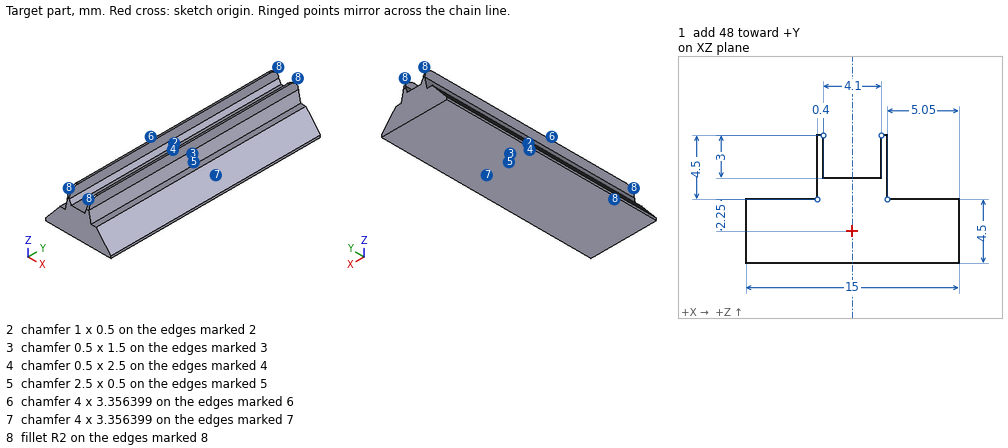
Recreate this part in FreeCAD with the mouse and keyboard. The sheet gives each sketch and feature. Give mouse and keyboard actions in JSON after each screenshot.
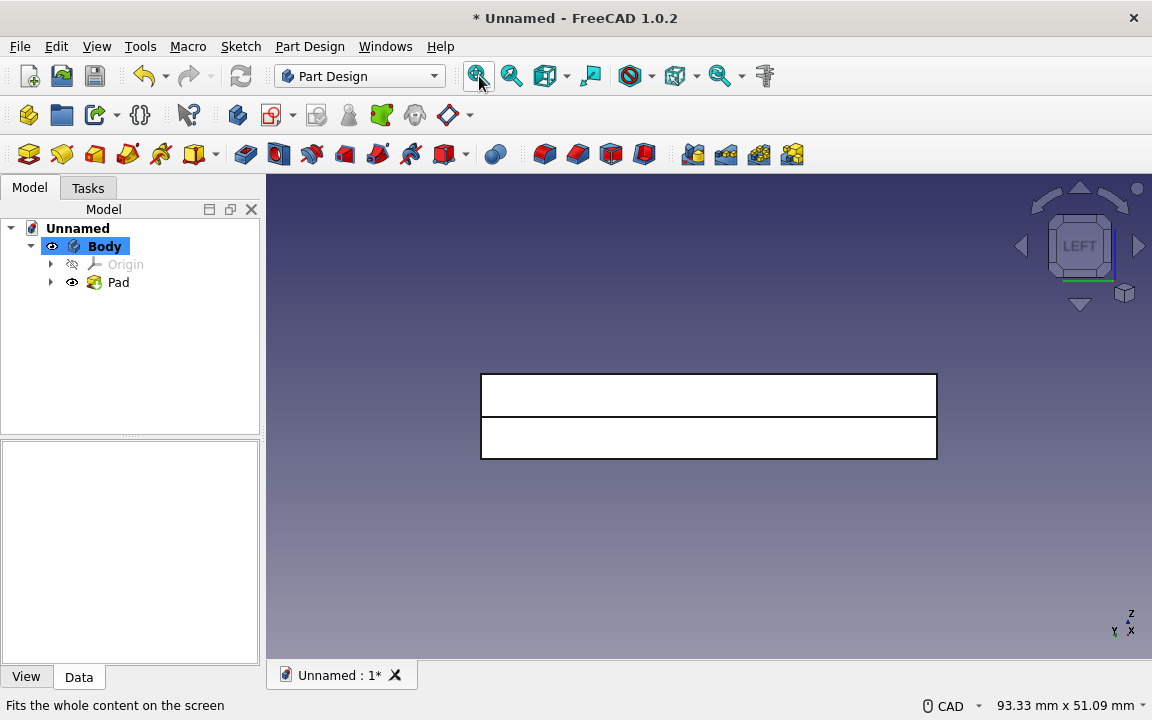
{"action": "key", "text": "v 3"}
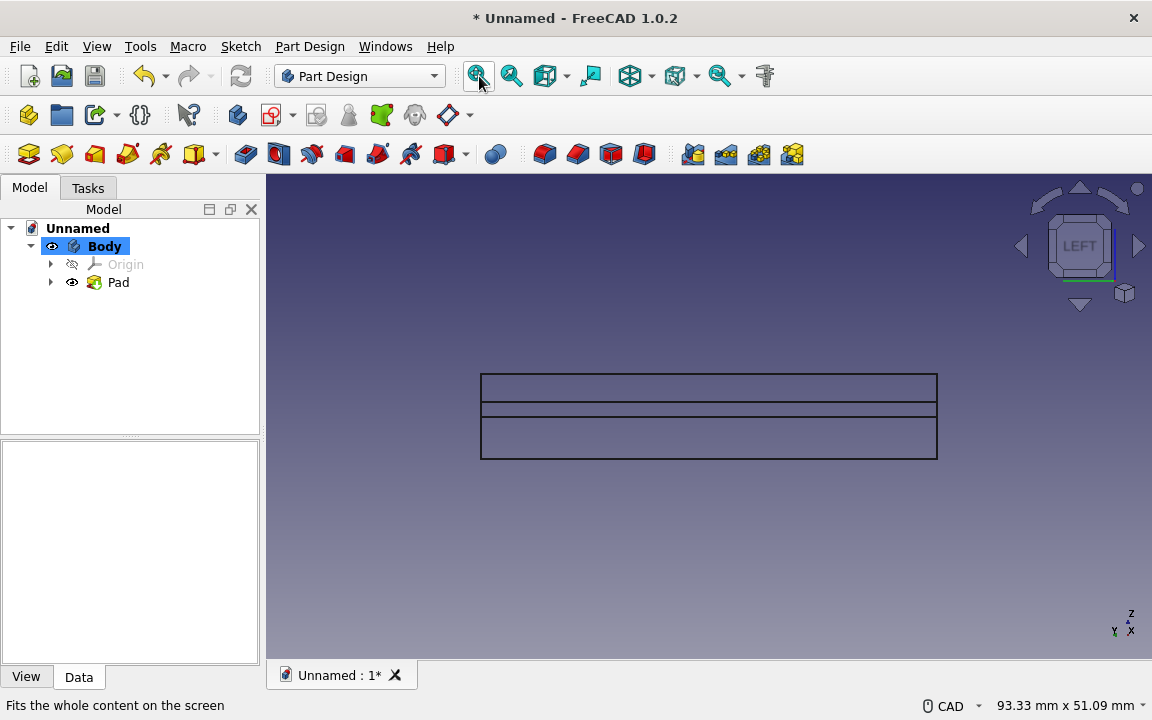
{"action": "key", "text": "0"}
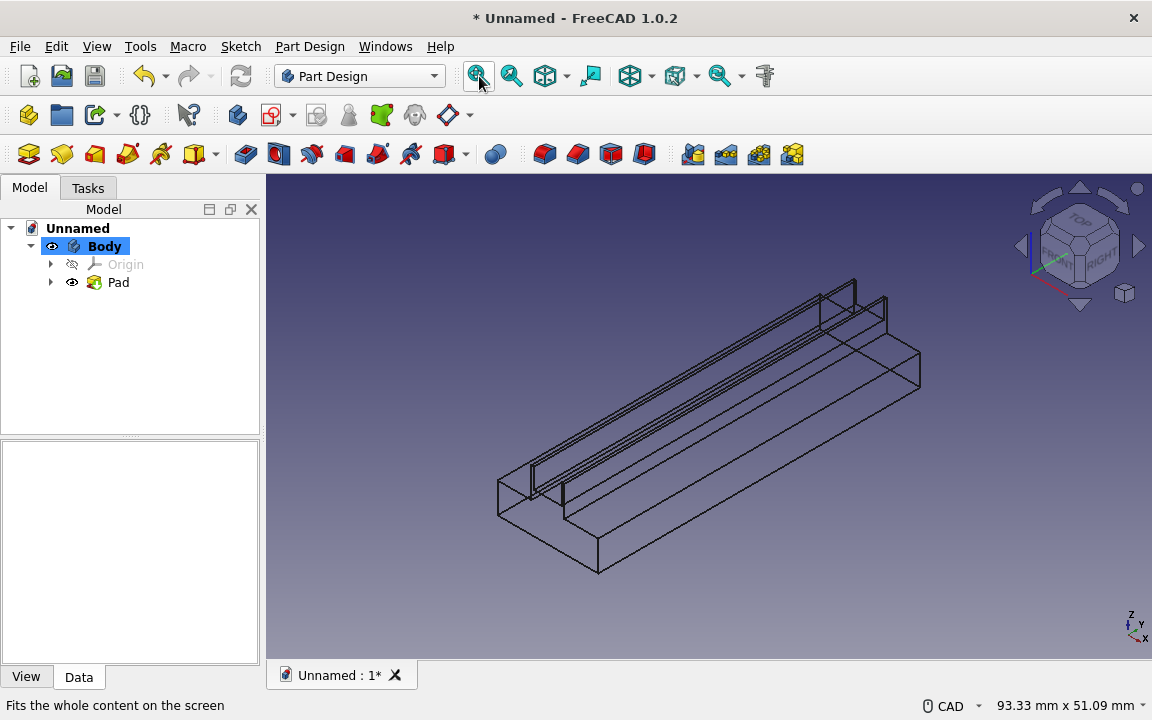
{"action": "left_click", "coordinate": [695, 396]}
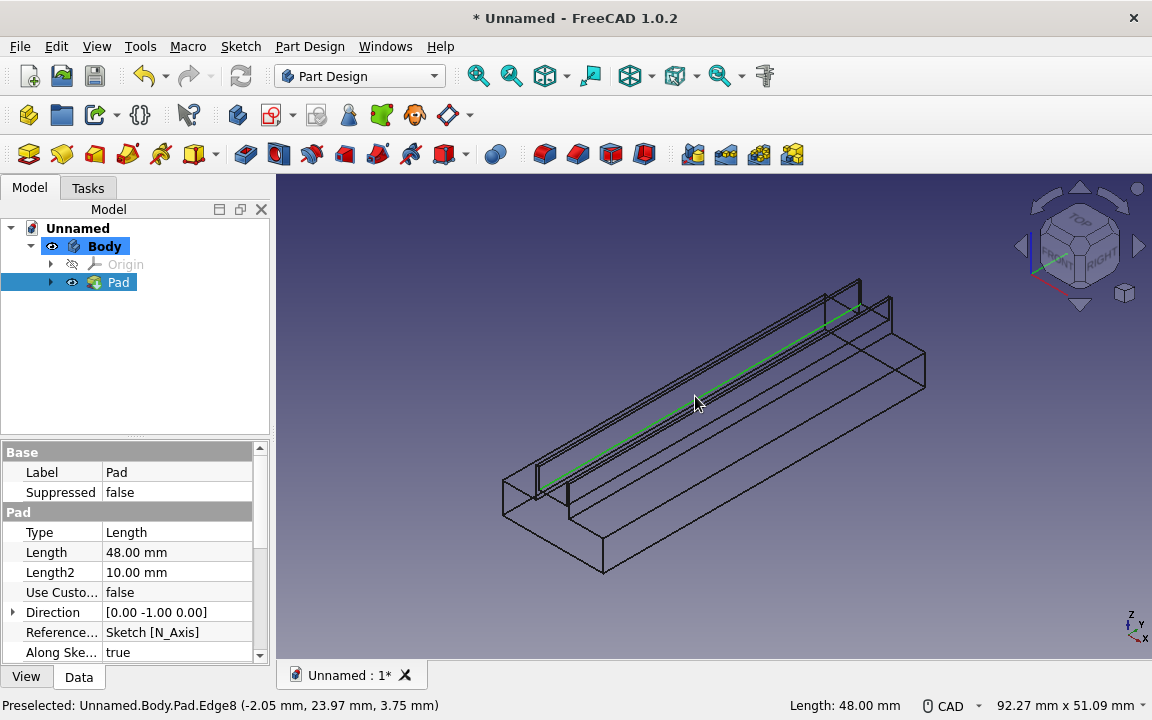
{"action": "key", "text": "v 1"}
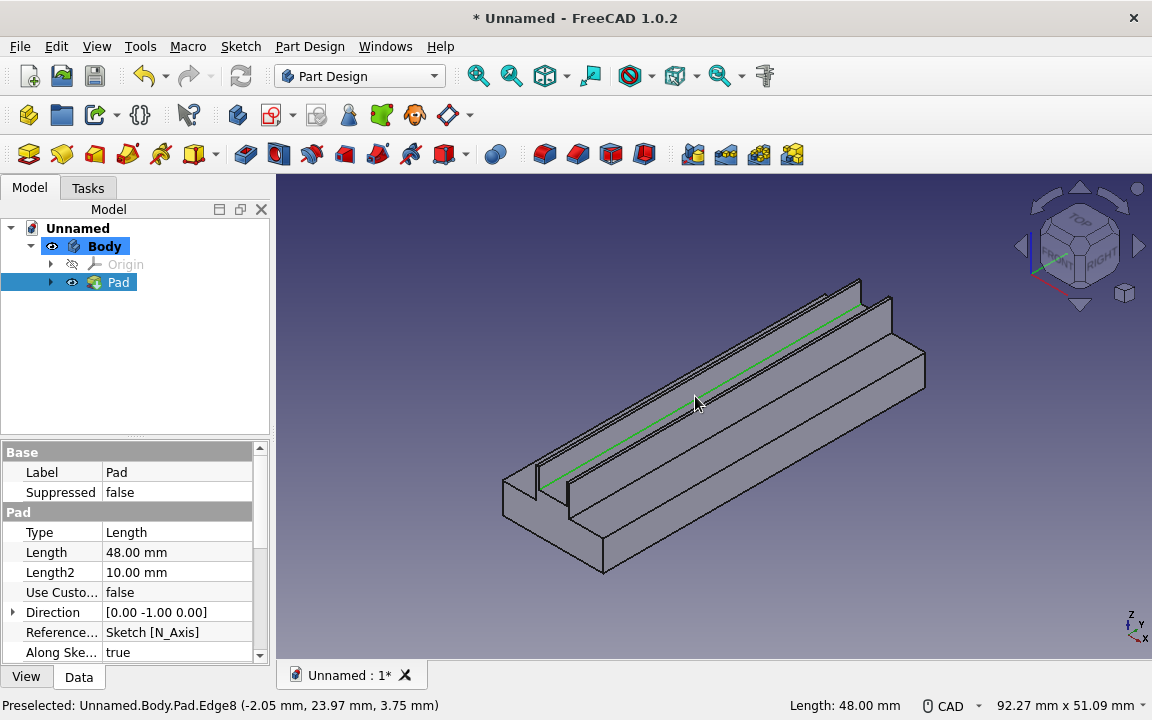
{"action": "left_click", "coordinate": [578, 154]}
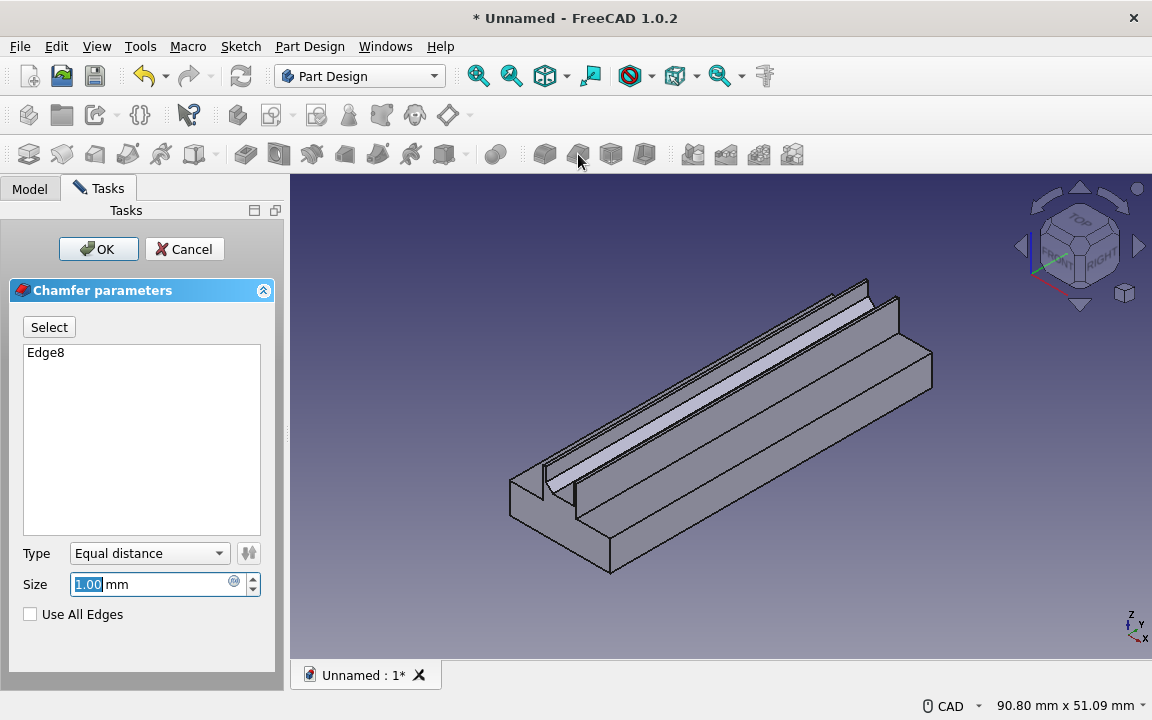
{"action": "type", "text": "1"}
{"action": "key", "text": "Tab"}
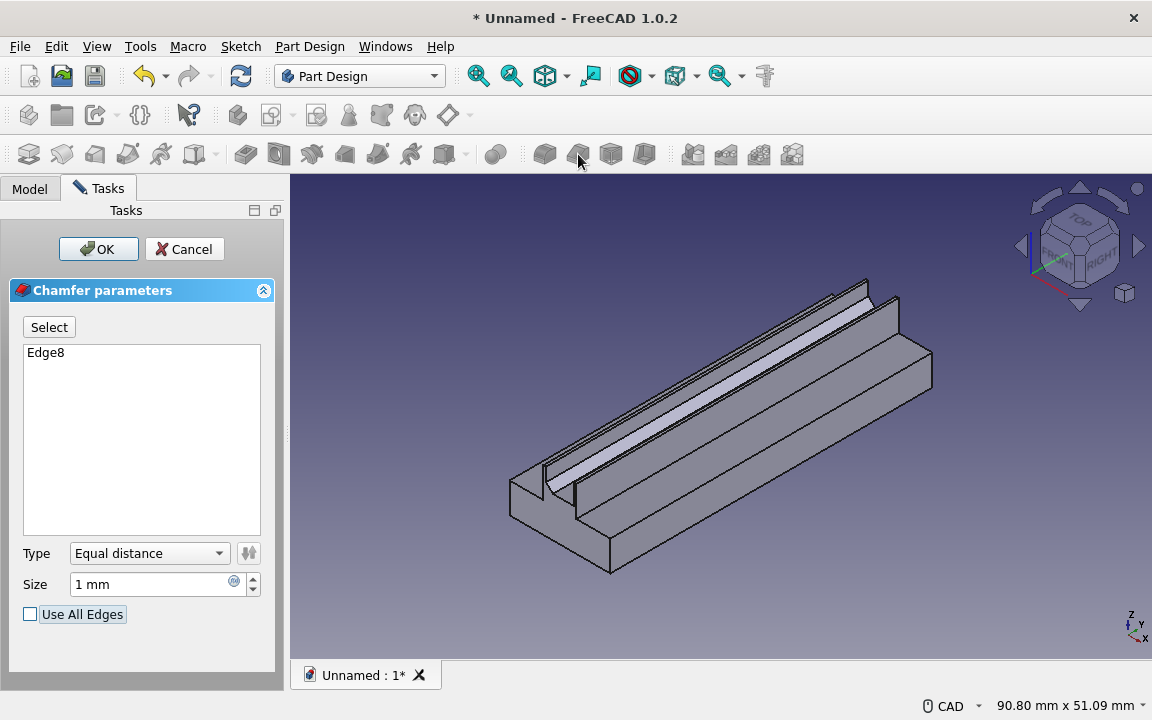
{"action": "left_click", "coordinate": [150, 554]}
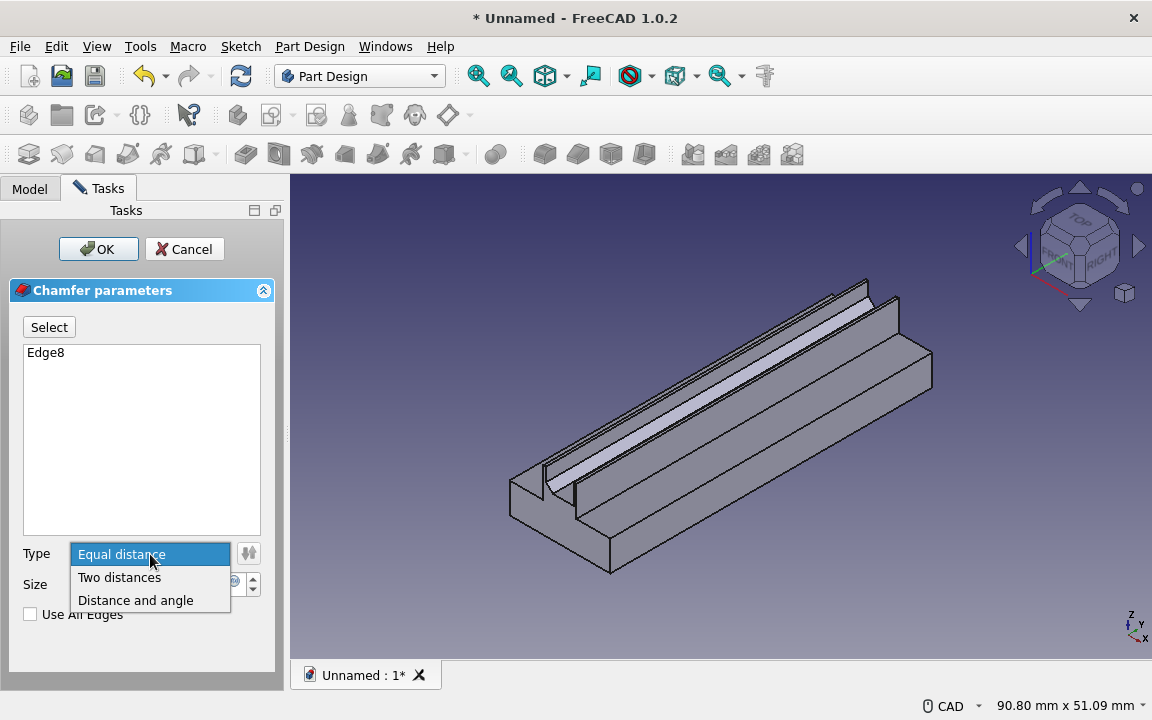
{"action": "left_click", "coordinate": [148, 578]}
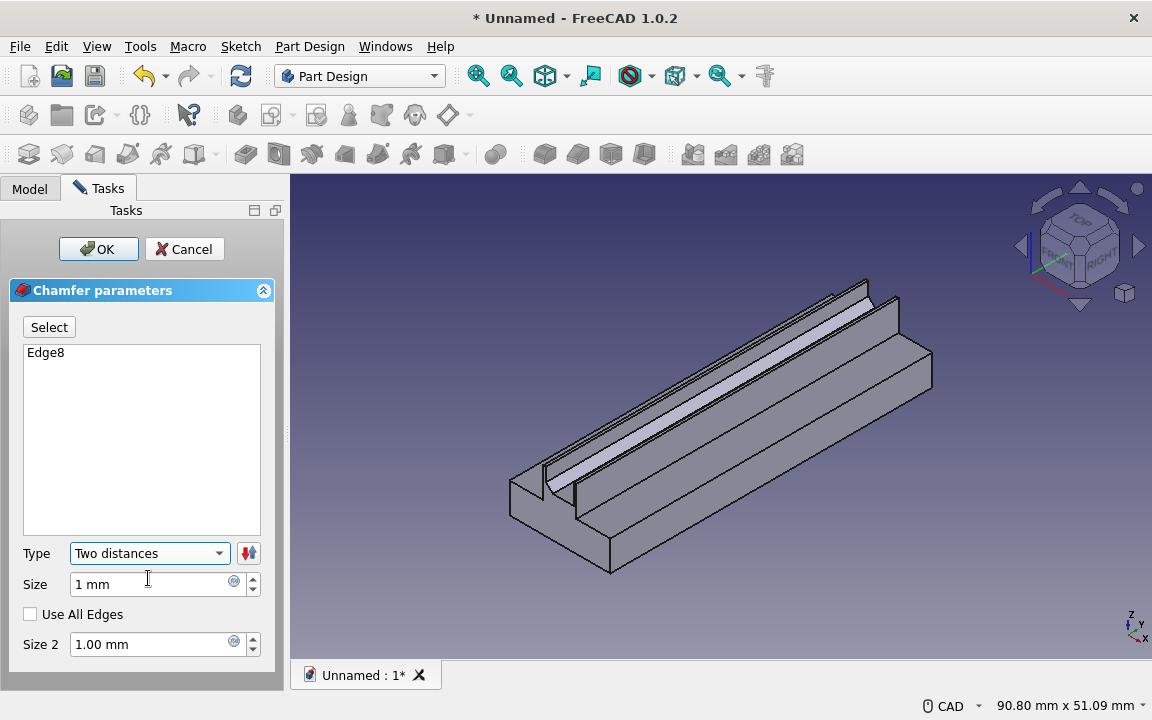
{"action": "triple_click", "coordinate": [158, 644]}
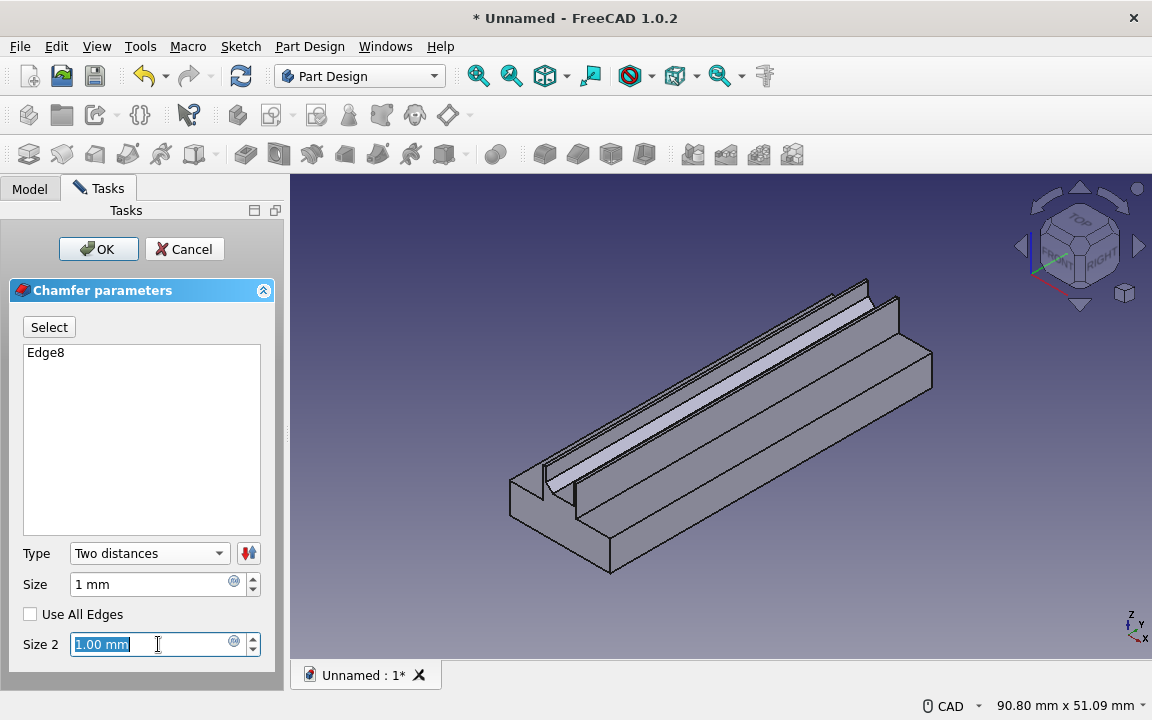
{"action": "type", "text": "0.5"}
{"action": "key", "text": "Tab"}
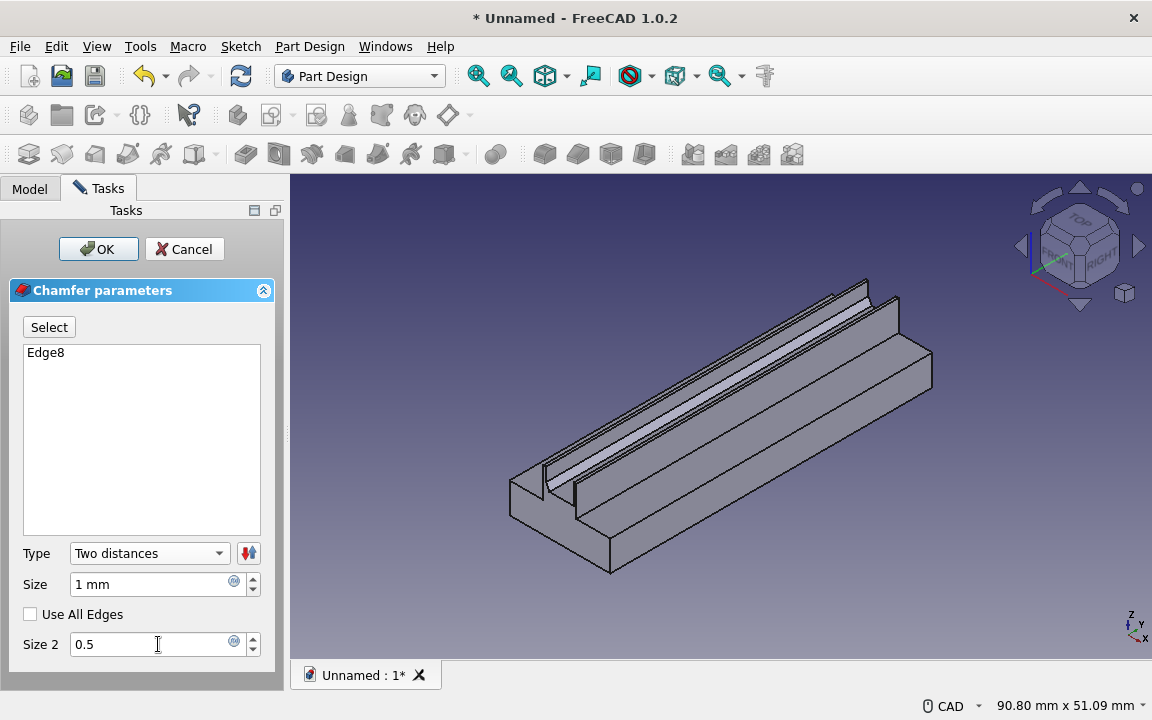
{"action": "left_click", "coordinate": [99, 249]}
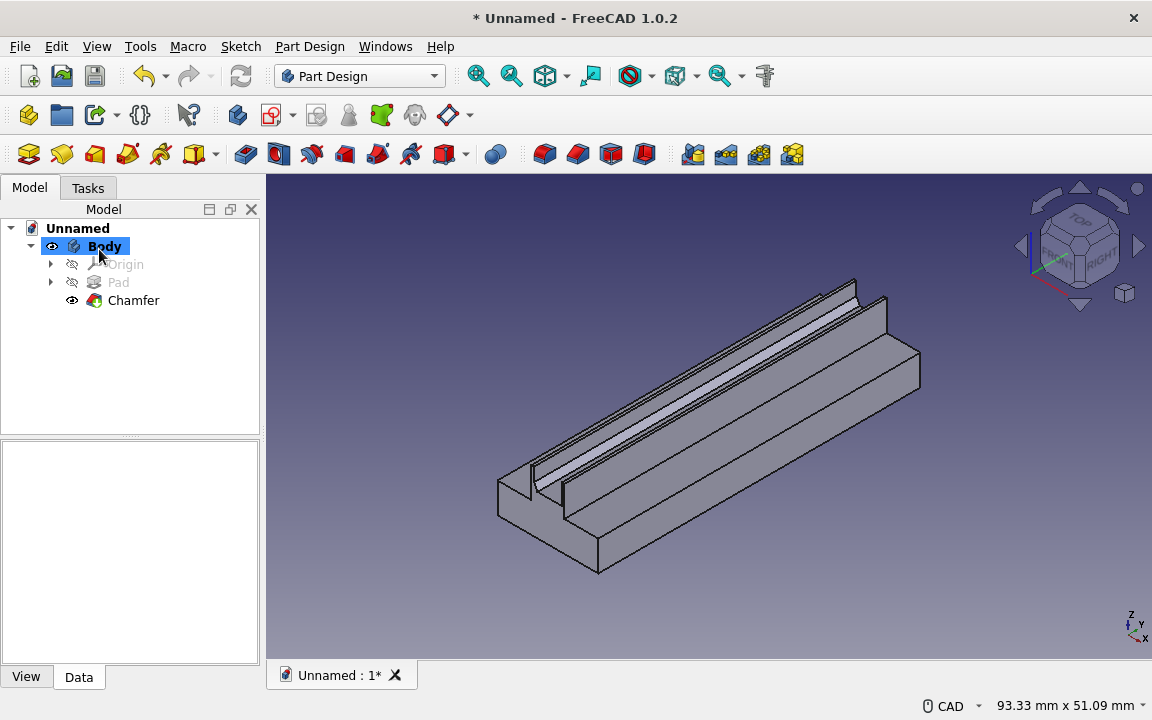
{"action": "key", "text": "2"}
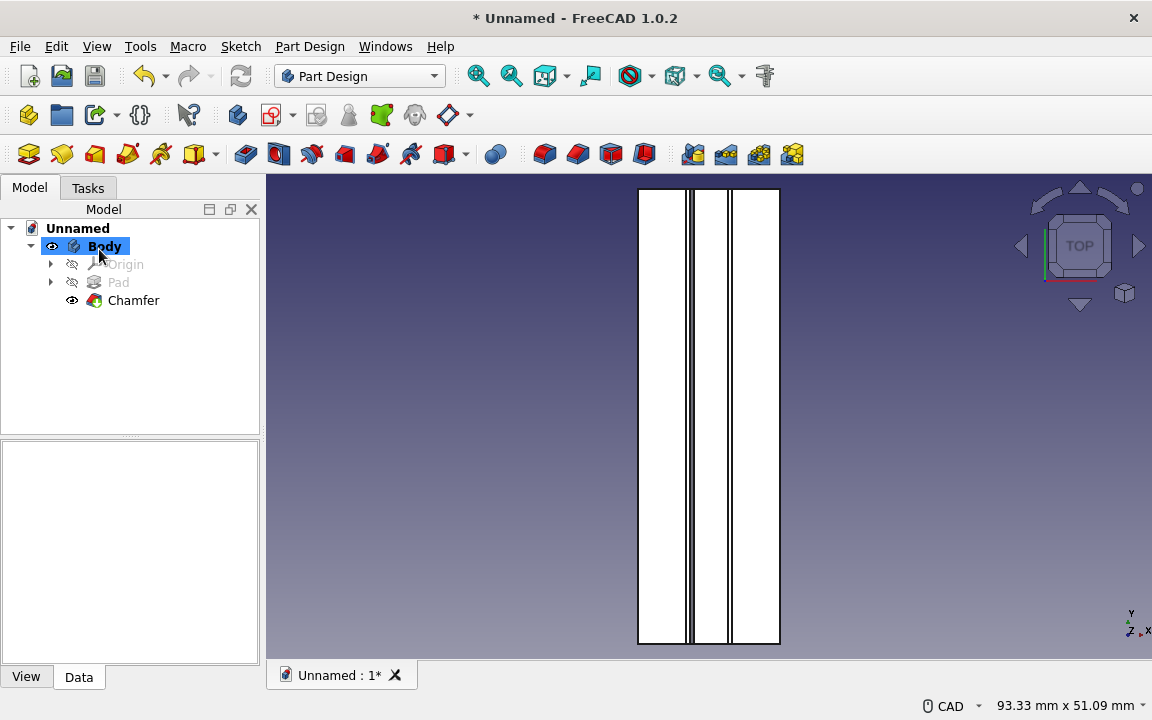
{"action": "key", "text": "0"}